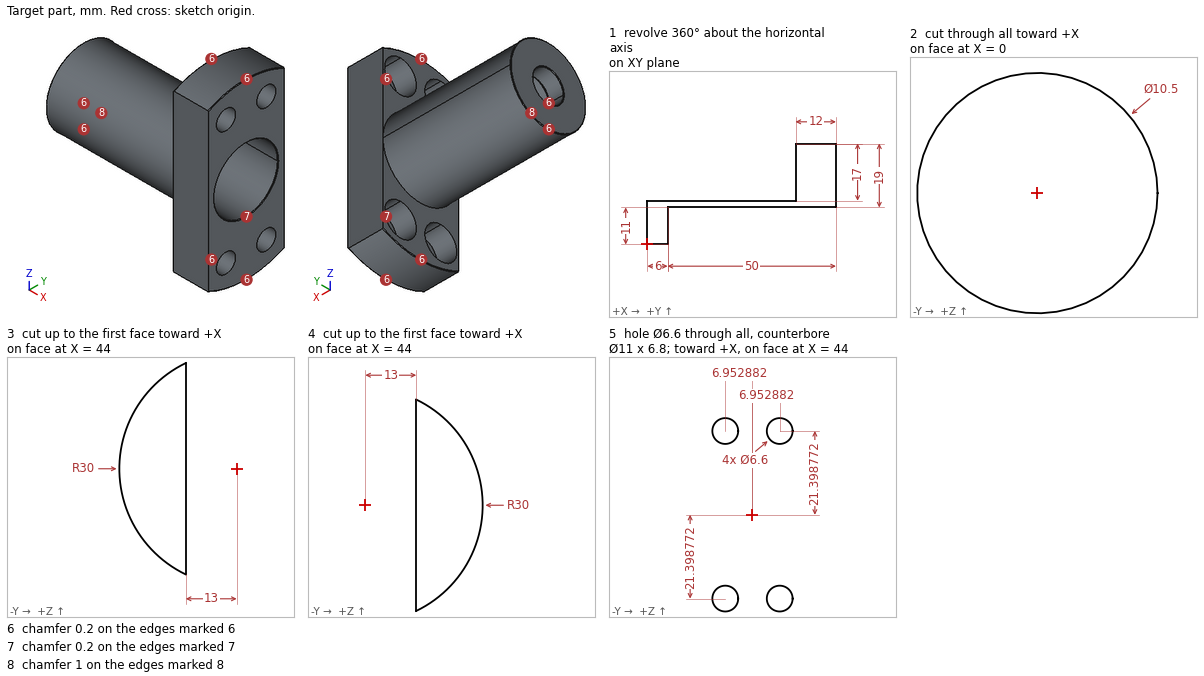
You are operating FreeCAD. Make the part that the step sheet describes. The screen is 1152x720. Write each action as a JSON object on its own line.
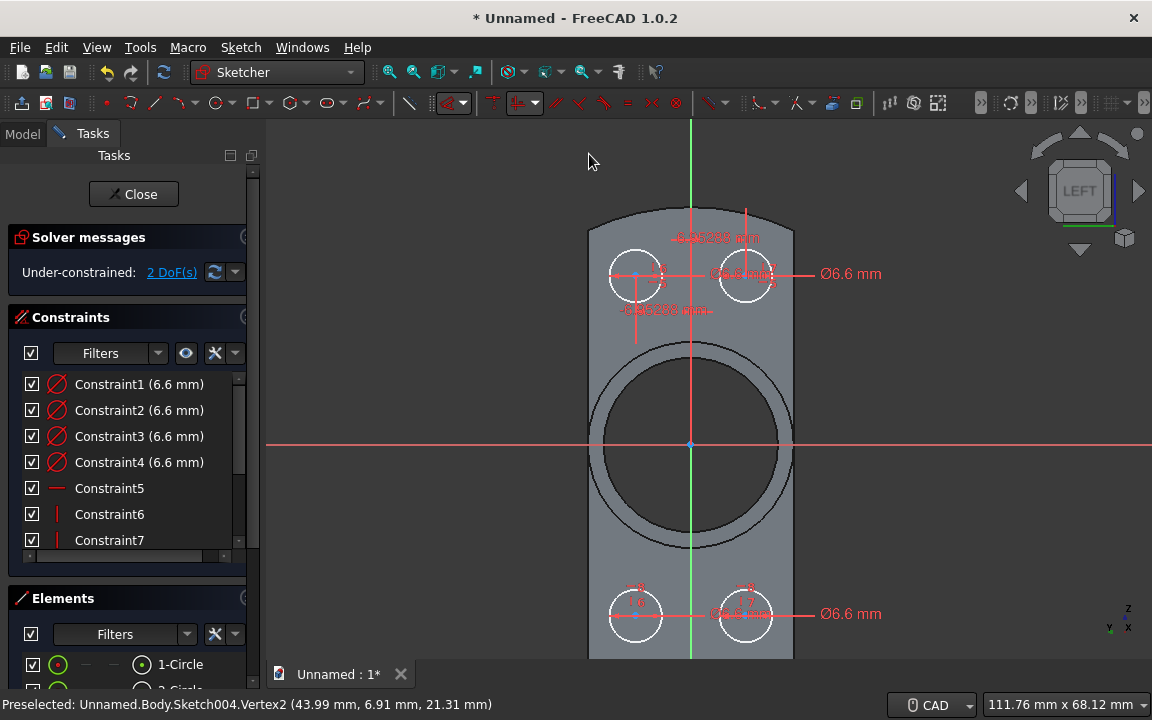
{"action": "left_click", "coordinate": [746, 276]}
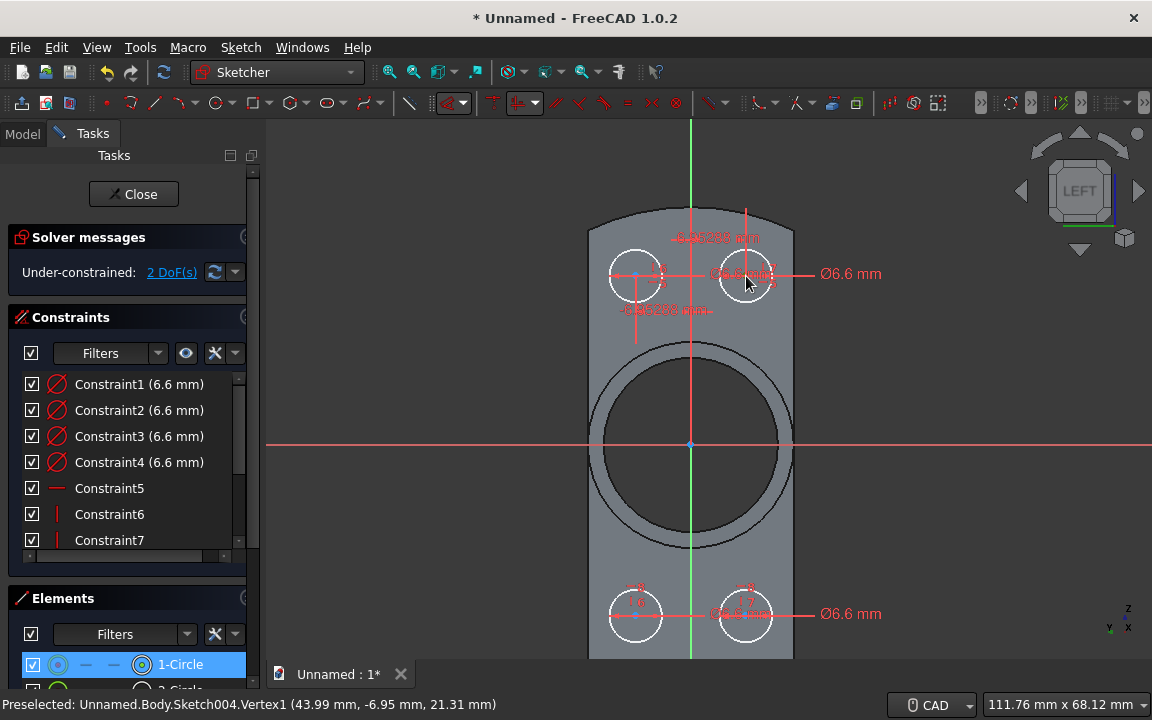
{"action": "left_click", "coordinate": [466, 104]}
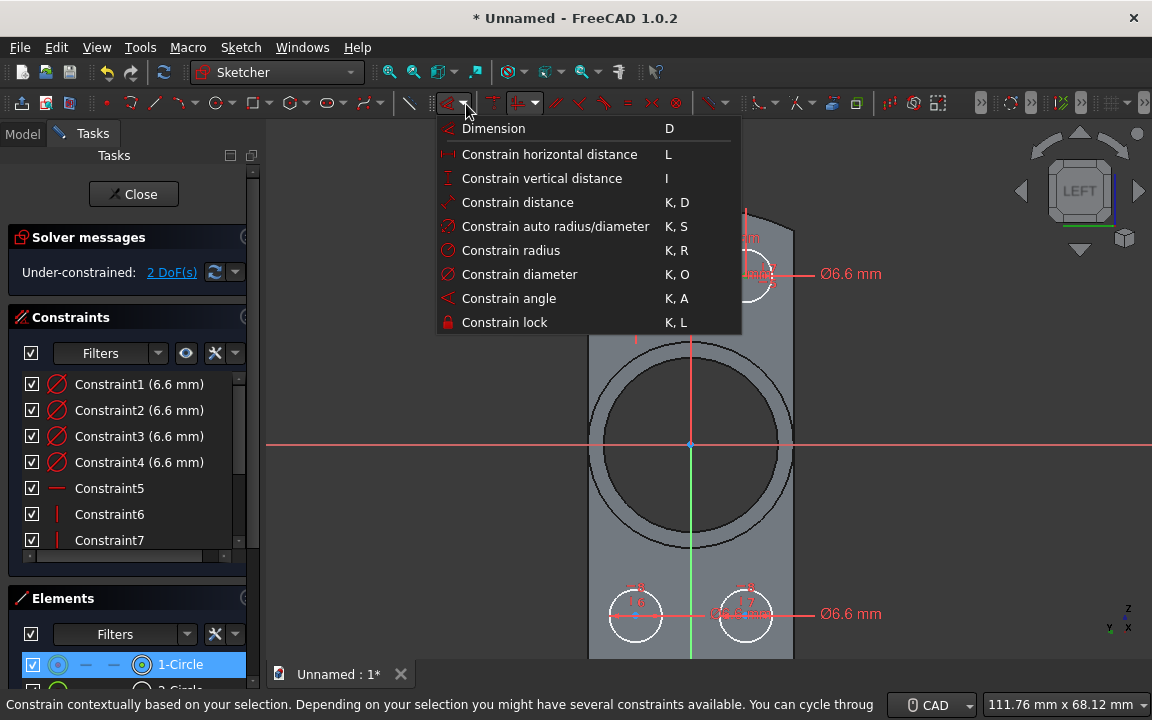
{"action": "left_click", "coordinate": [589, 178]}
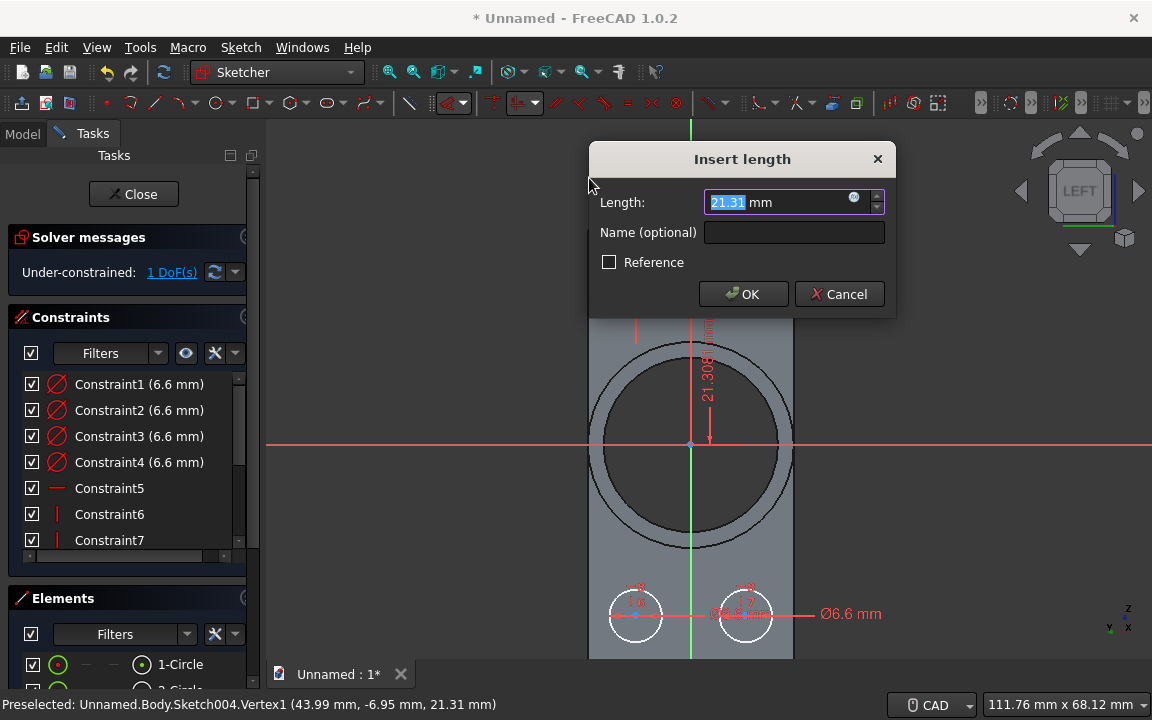
{"action": "type", "text": "21.398772"}
{"action": "key", "text": "Return"}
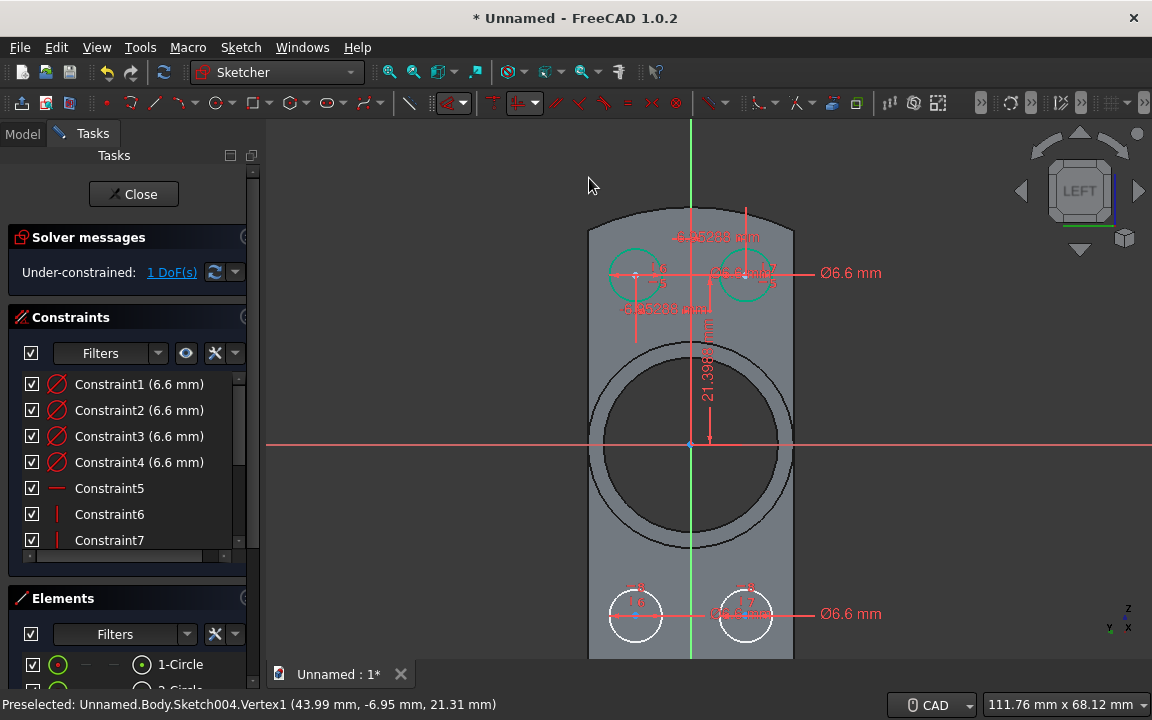
{"action": "left_click", "coordinate": [636, 616]}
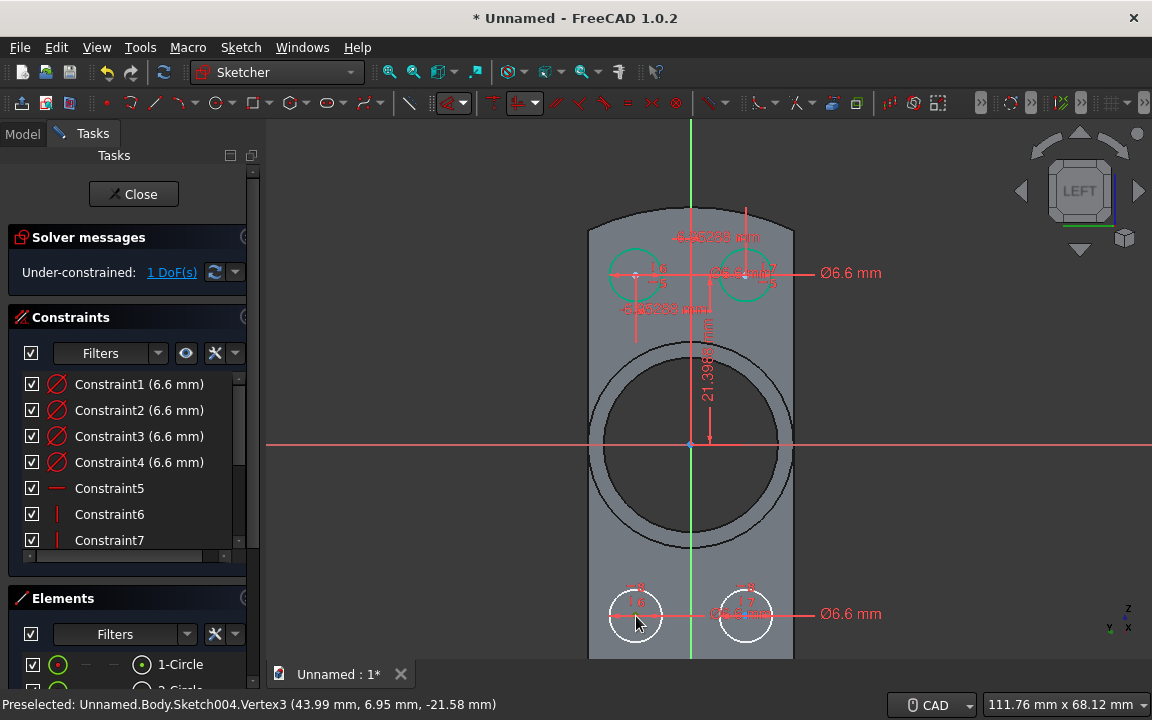
{"action": "key", "text": "i"}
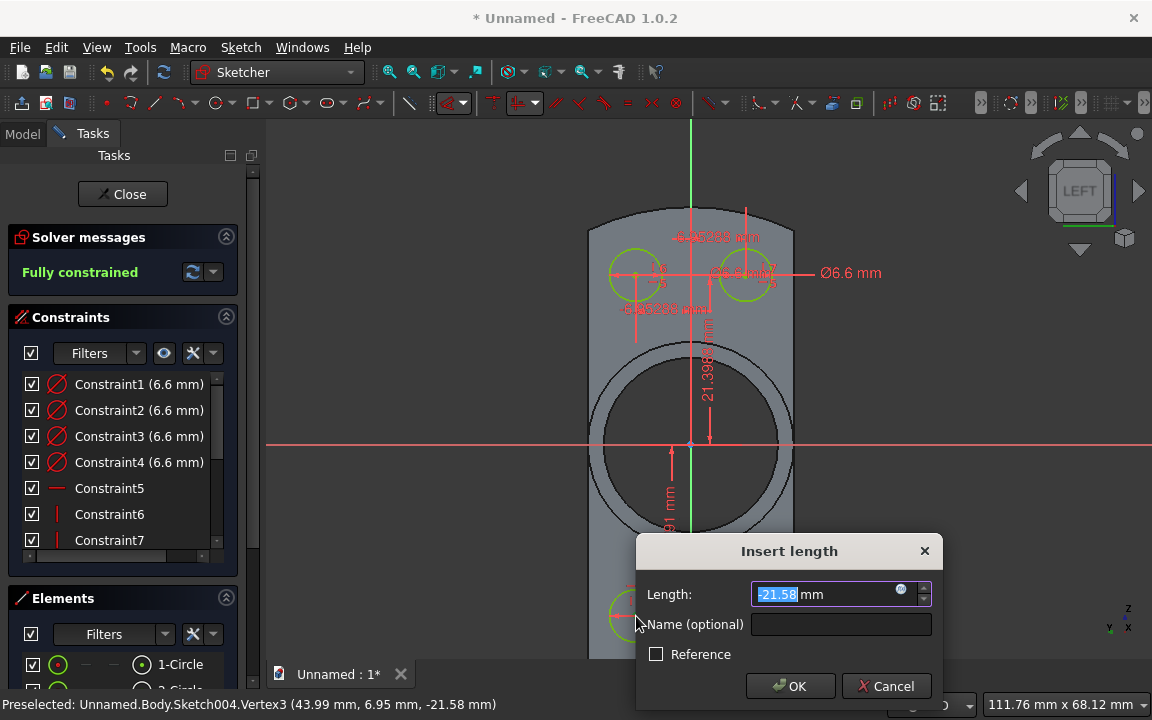
{"action": "type", "text": "-21.398772"}
{"action": "key", "text": "Return"}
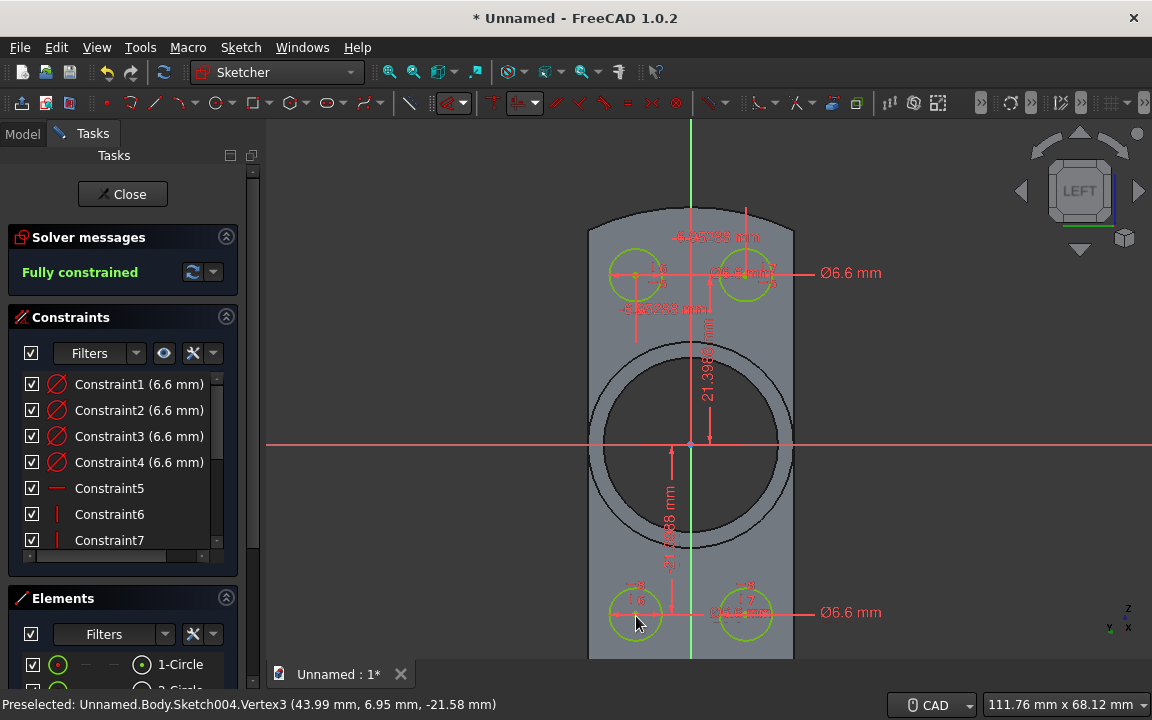
{"action": "left_click", "coordinate": [123, 194]}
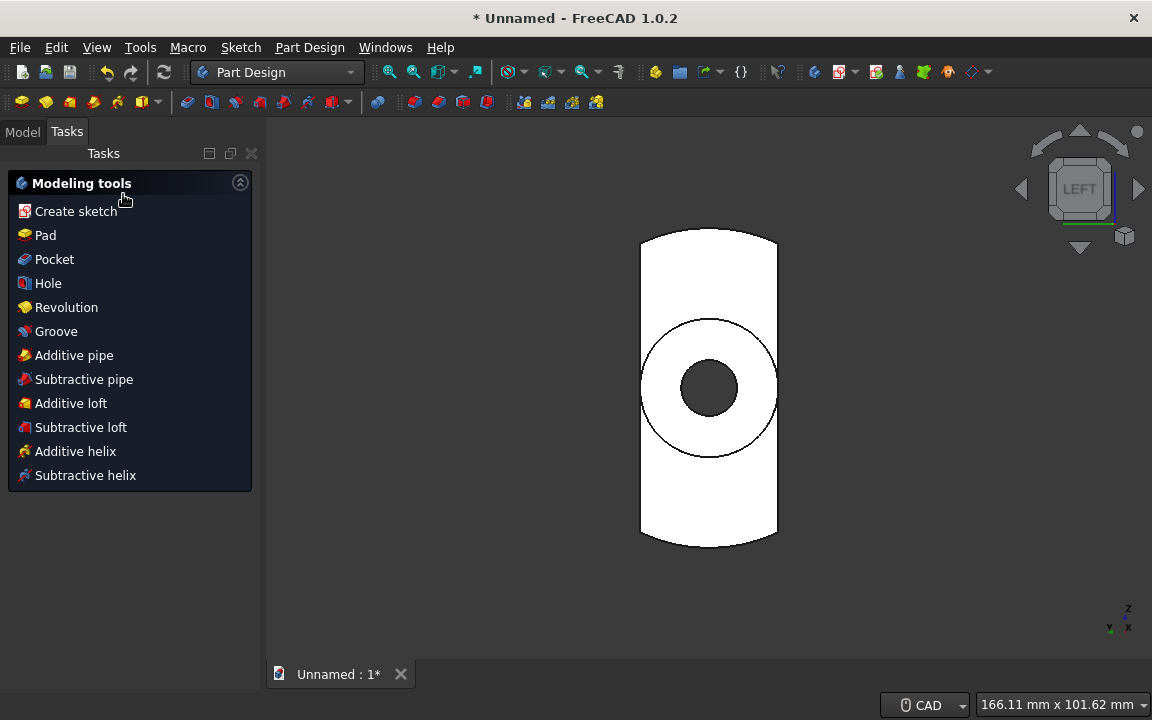
{"action": "left_click", "coordinate": [212, 102]}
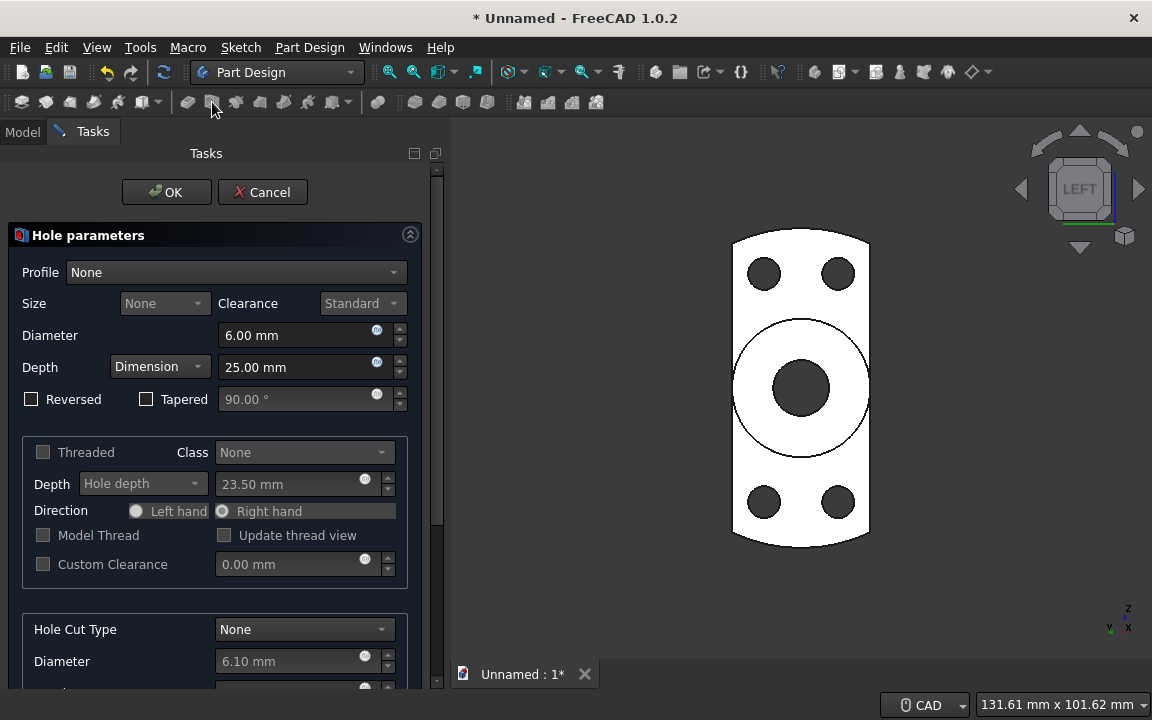
{"action": "triple_click", "coordinate": [305, 335]}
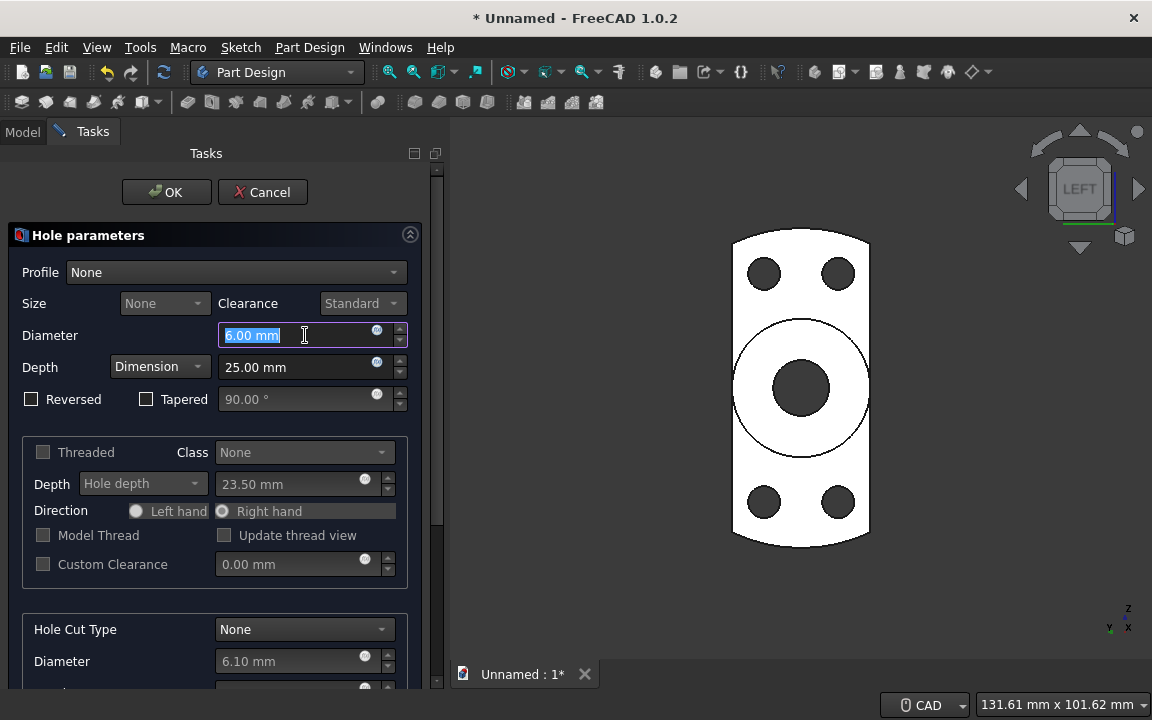
{"action": "type", "text": "6.6"}
{"action": "key", "text": "Tab"}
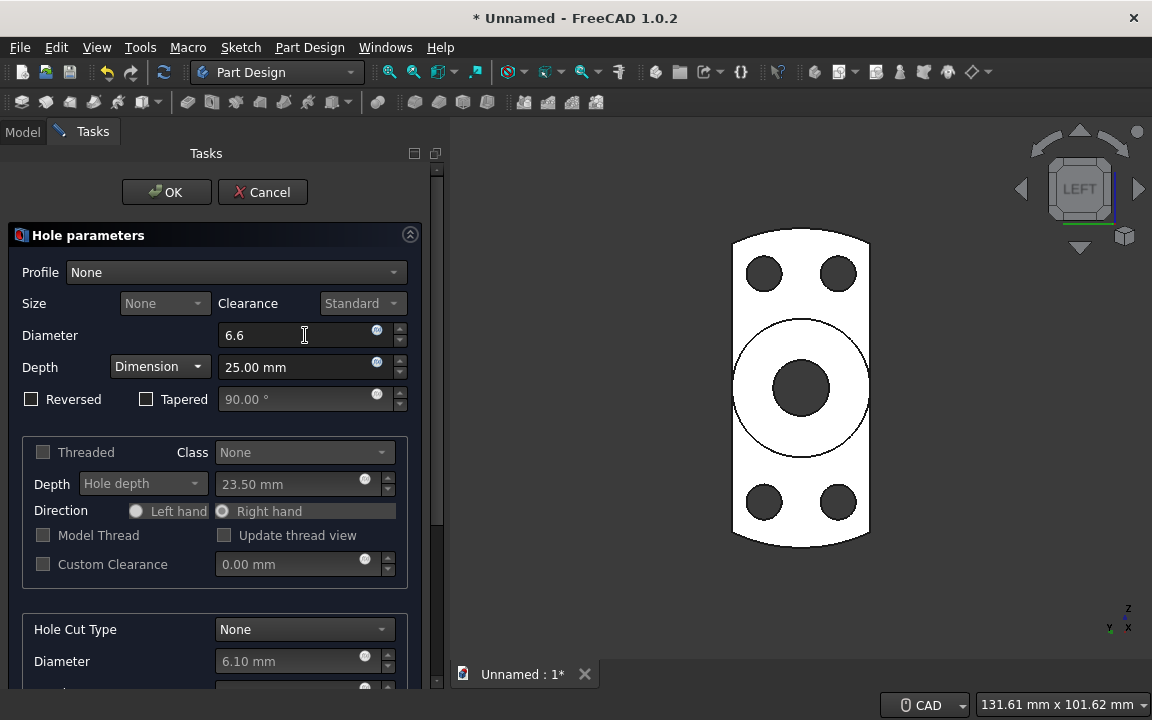
{"action": "left_click", "coordinate": [161, 366]}